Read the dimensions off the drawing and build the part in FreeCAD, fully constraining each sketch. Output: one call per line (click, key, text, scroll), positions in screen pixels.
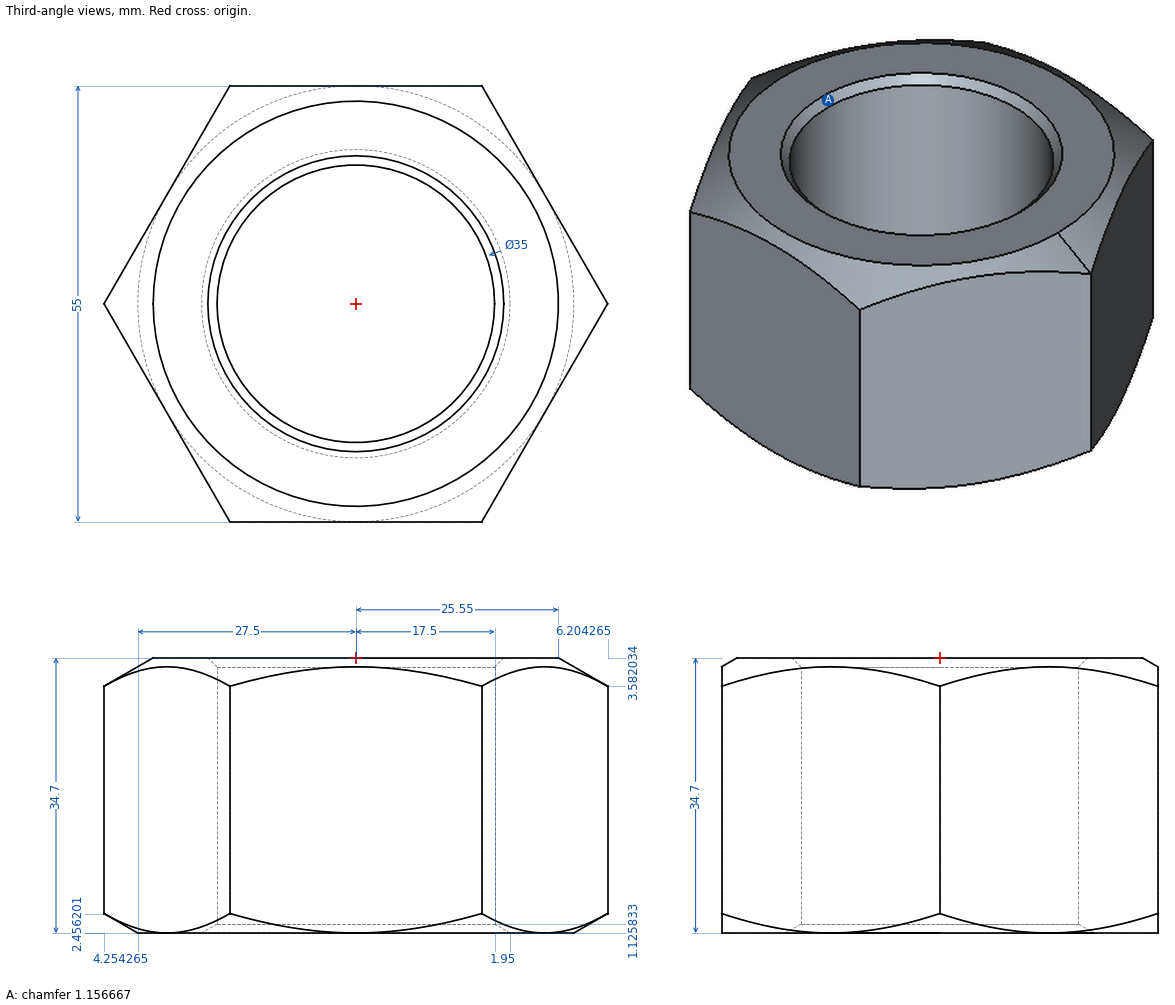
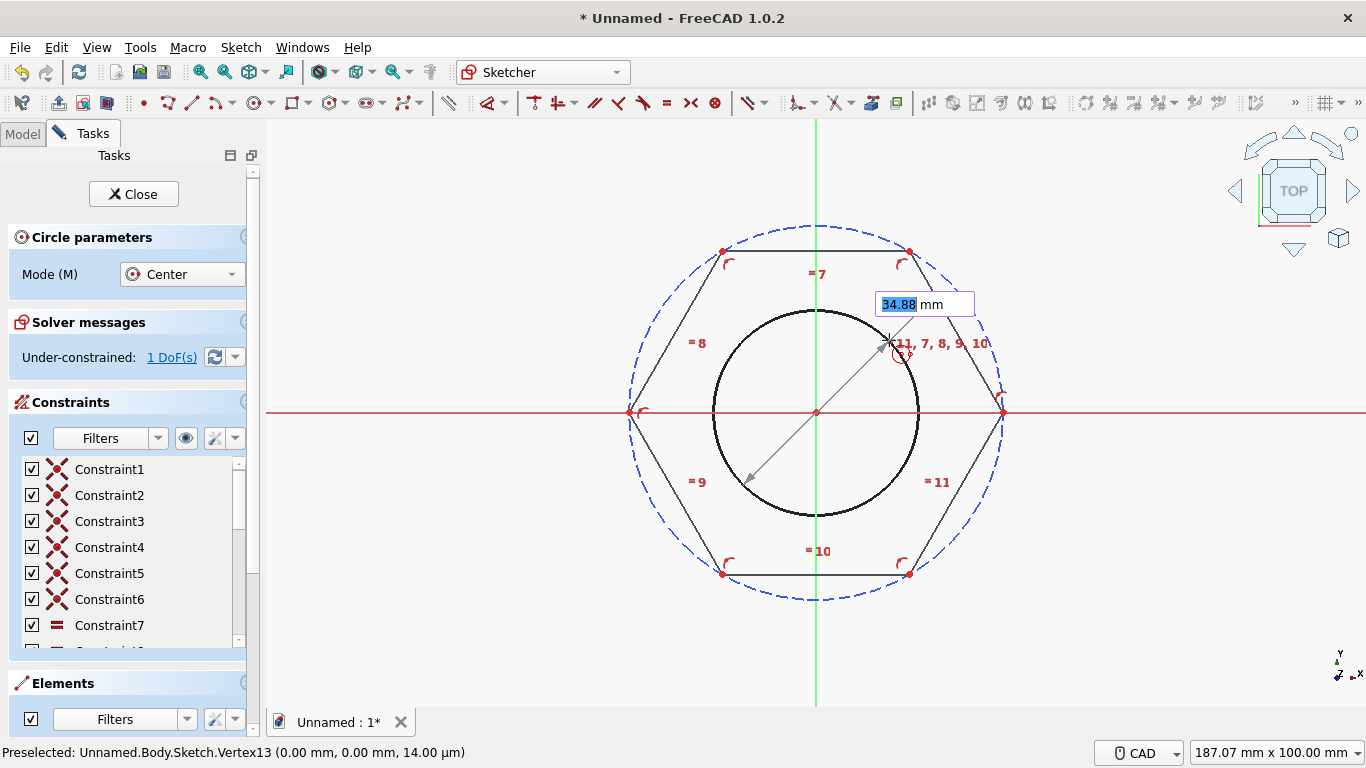
text(35)
key(Return)
key(Escape)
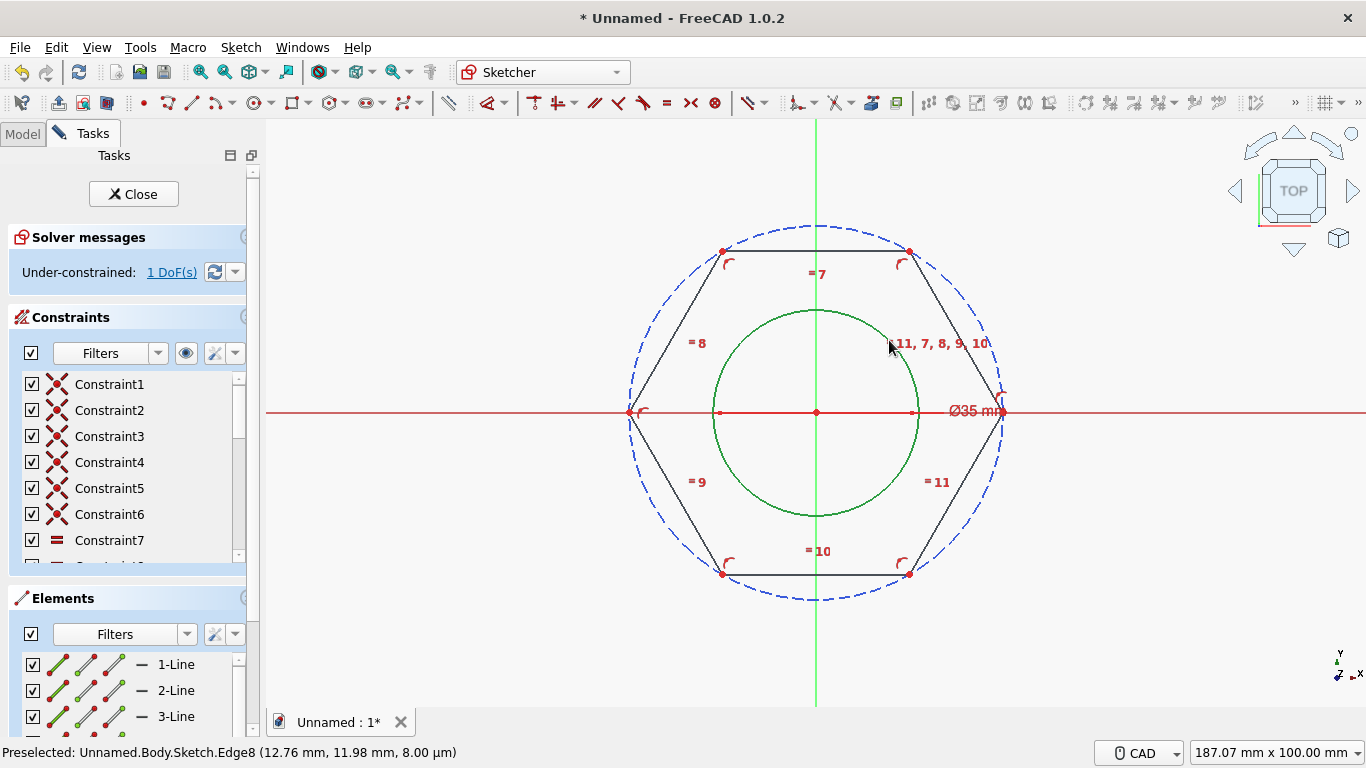
click(722, 575)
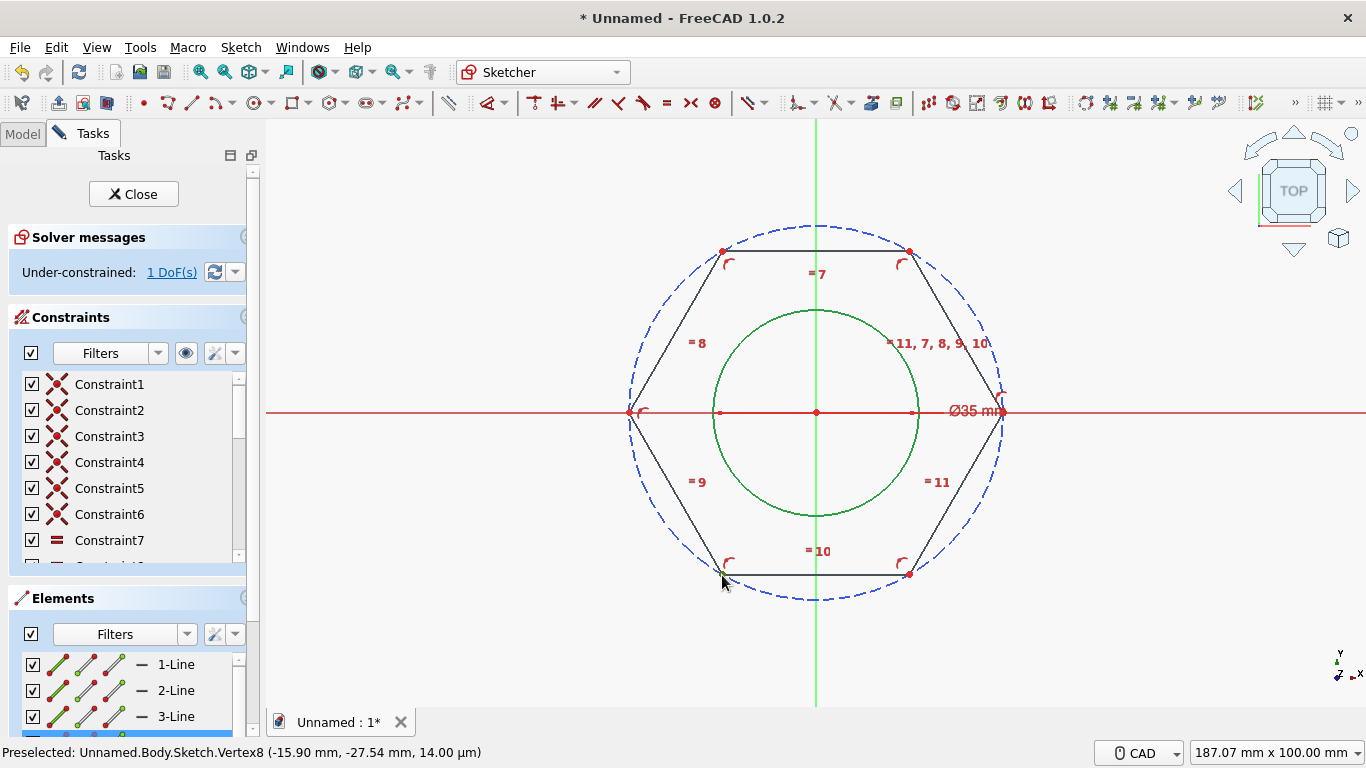
click(910, 251)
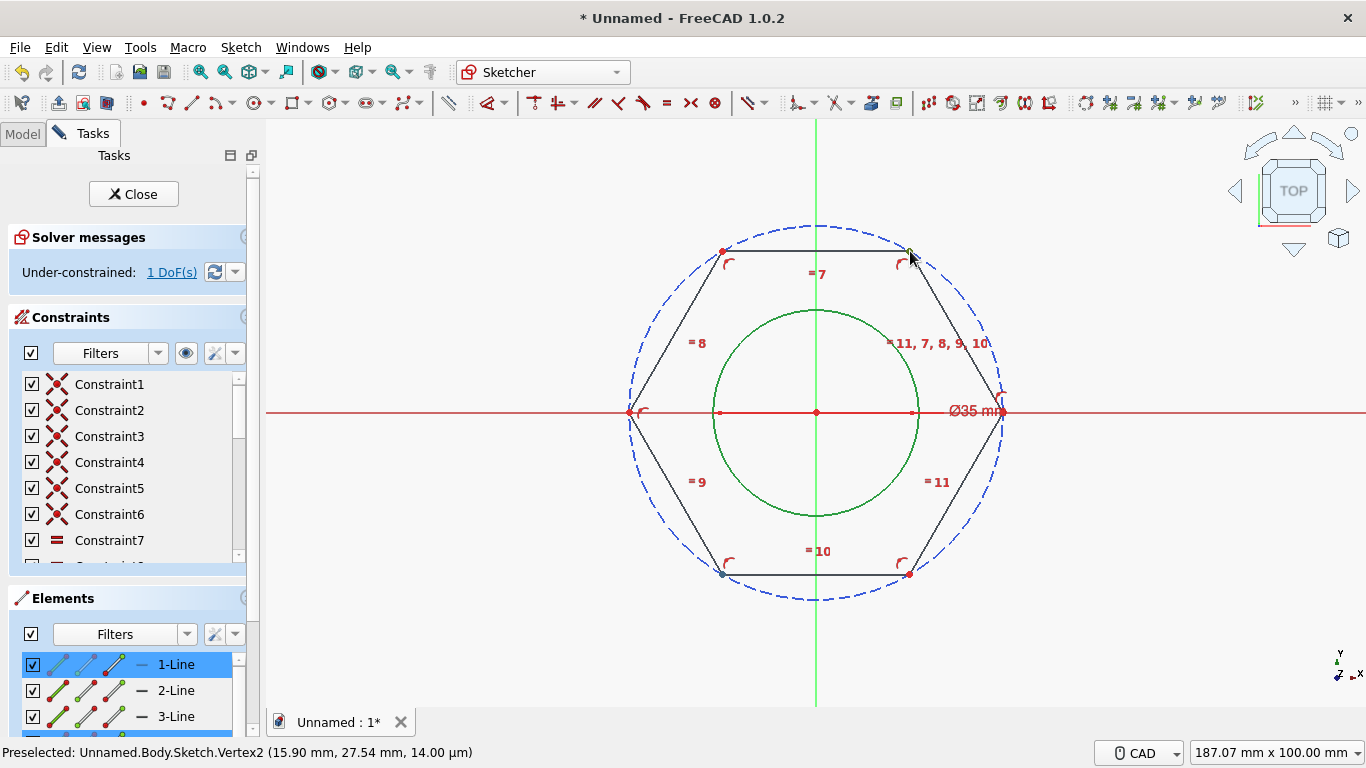
key(i)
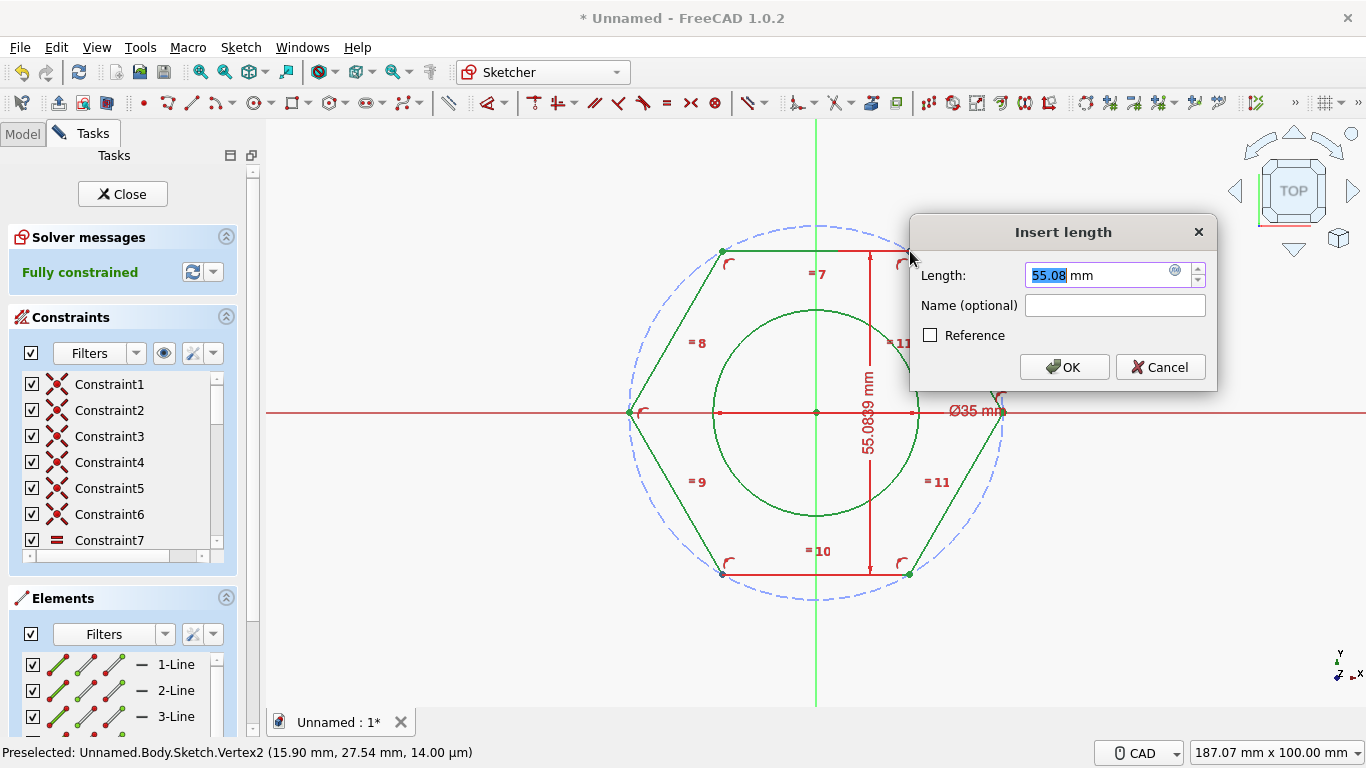
text(55)
key(Return)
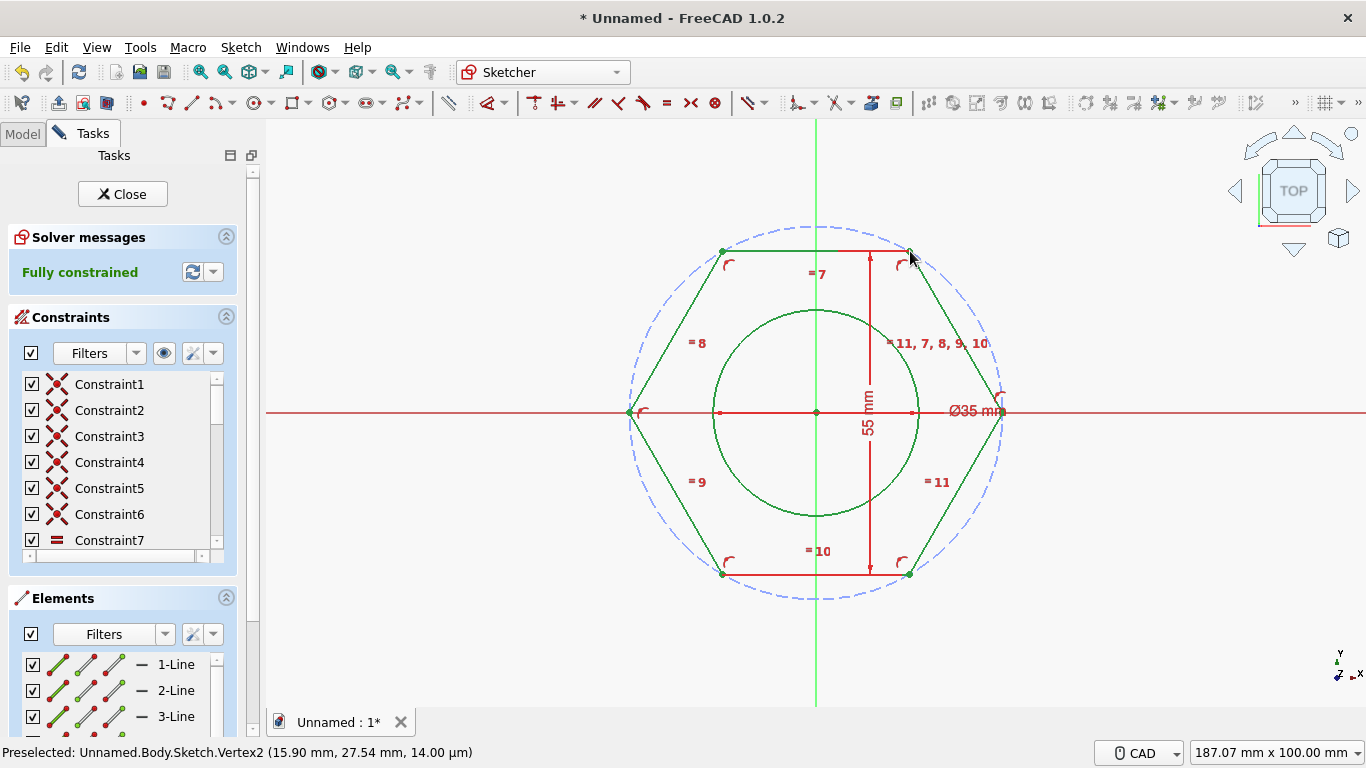
click(123, 194)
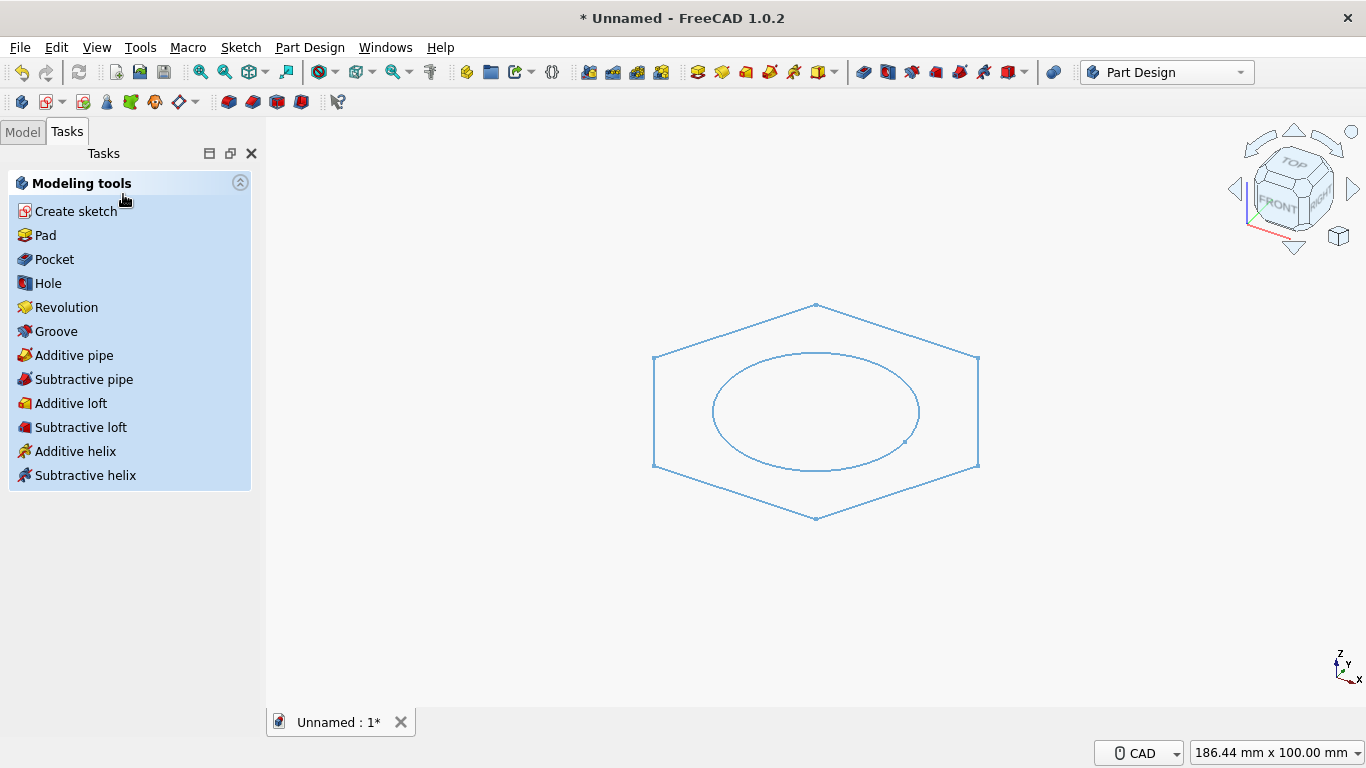
click(698, 72)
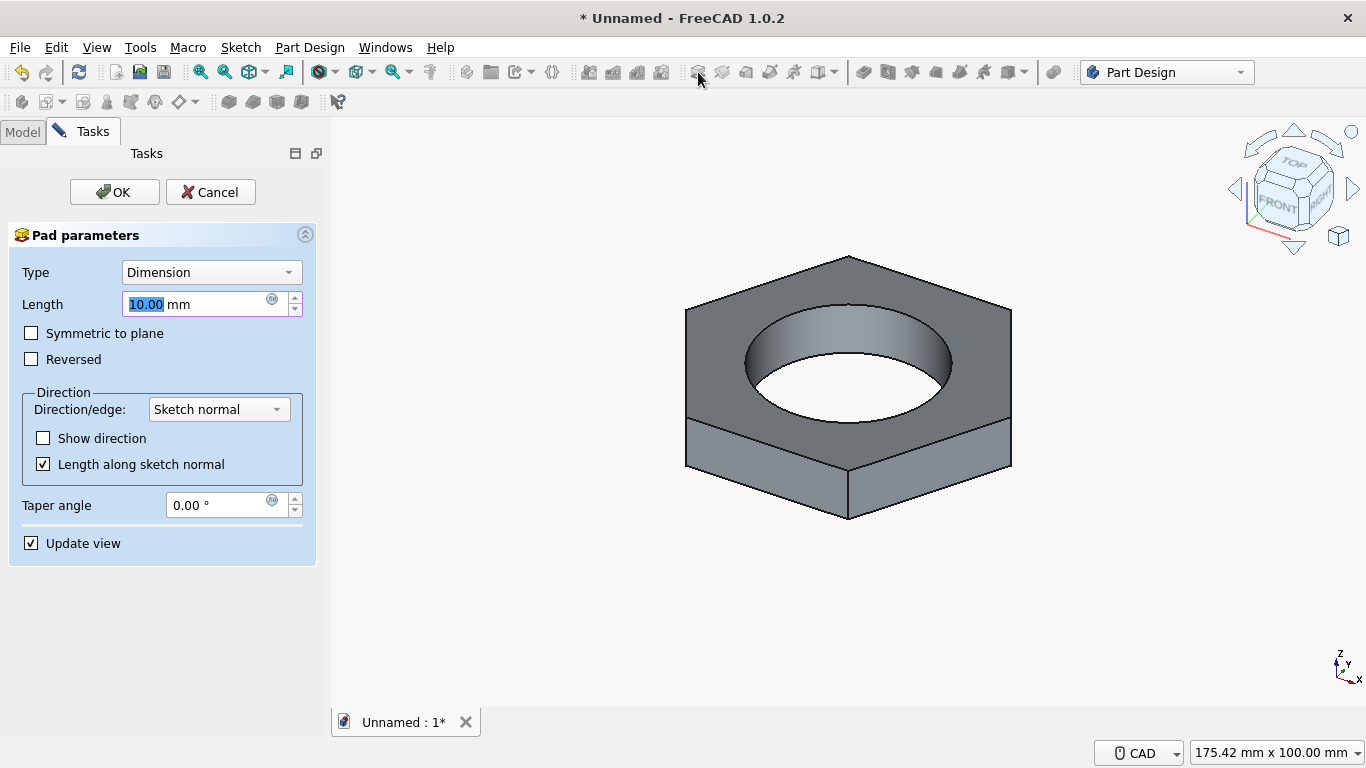
text(34.7)
key(Tab)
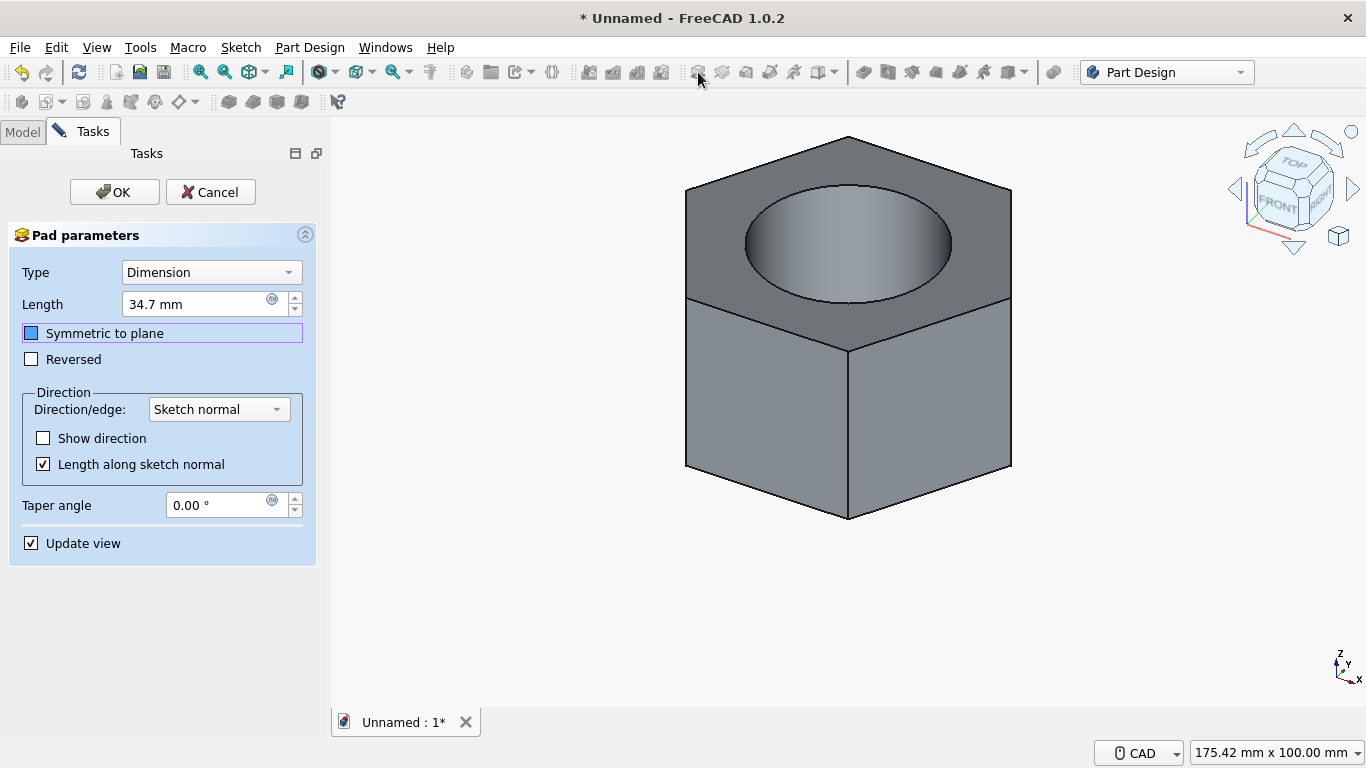
click(30, 359)